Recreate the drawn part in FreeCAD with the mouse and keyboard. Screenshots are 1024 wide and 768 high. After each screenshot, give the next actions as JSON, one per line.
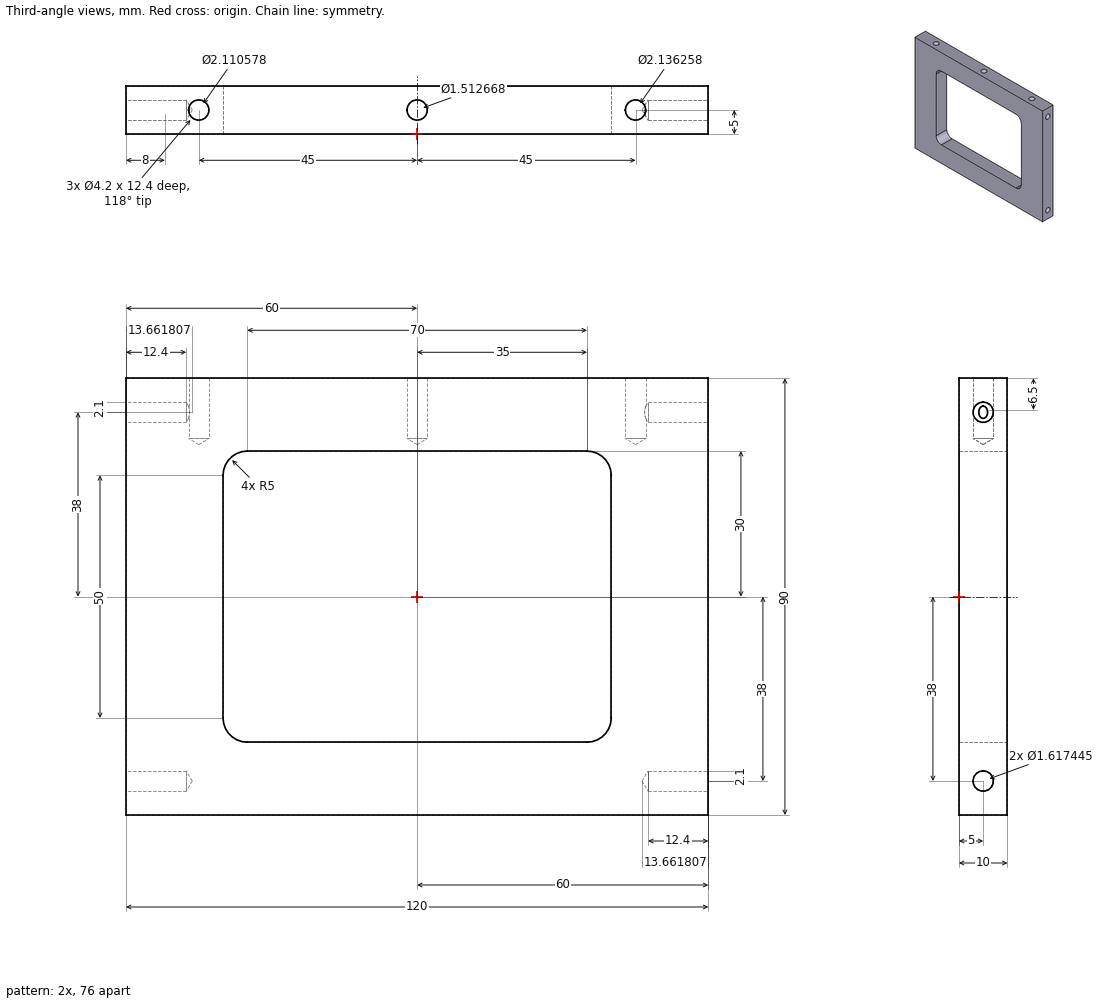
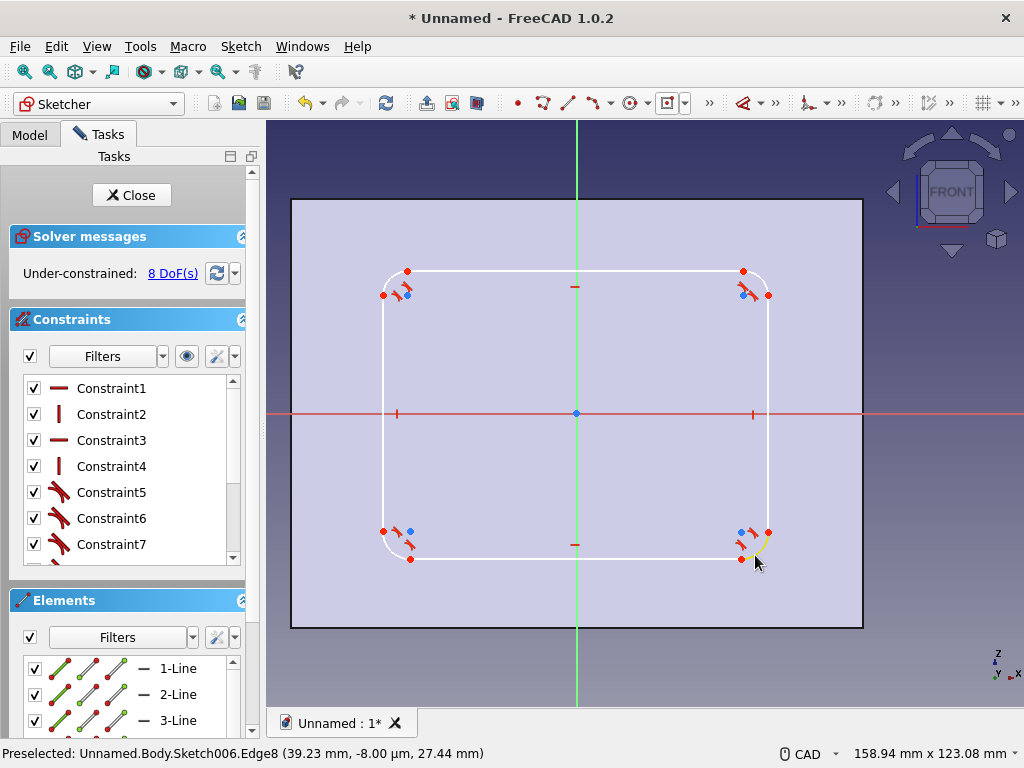
{"action": "left_click", "coordinate": [396, 274]}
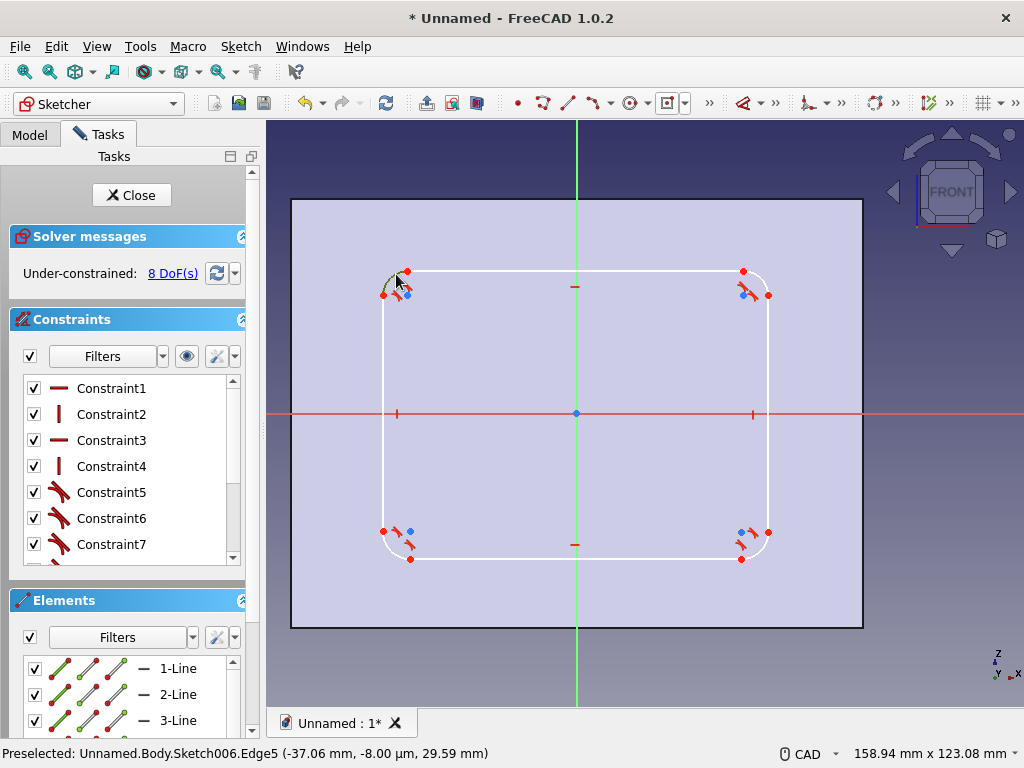
{"action": "left_click", "coordinate": [386, 544]}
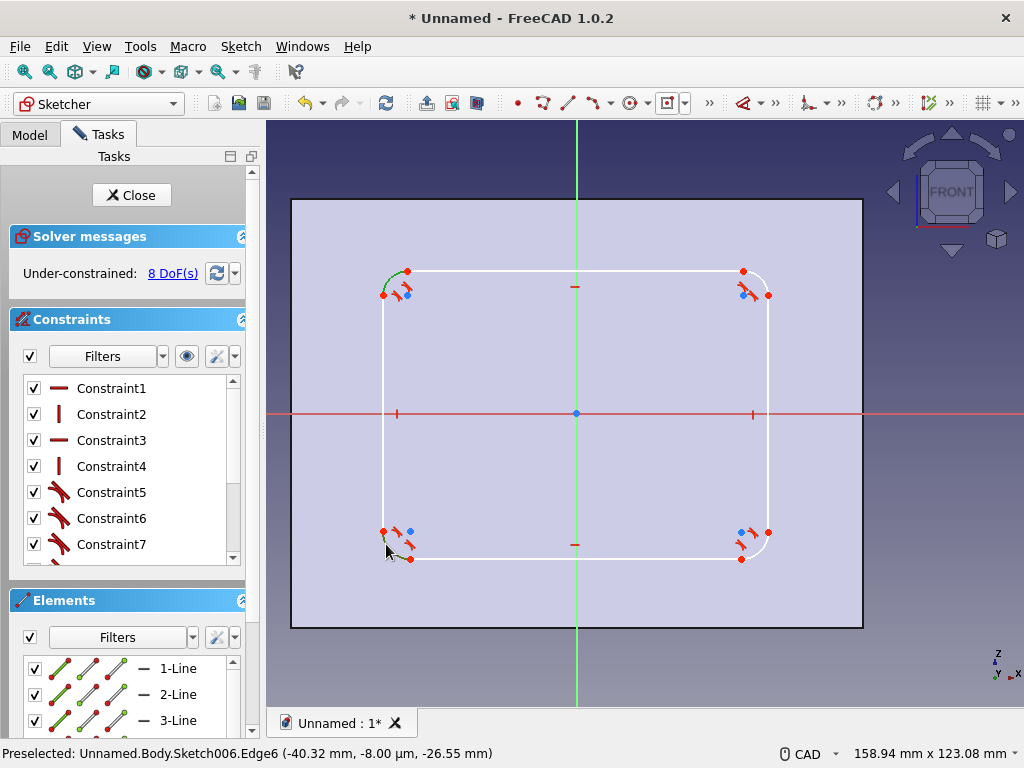
{"action": "left_click", "coordinate": [754, 556]}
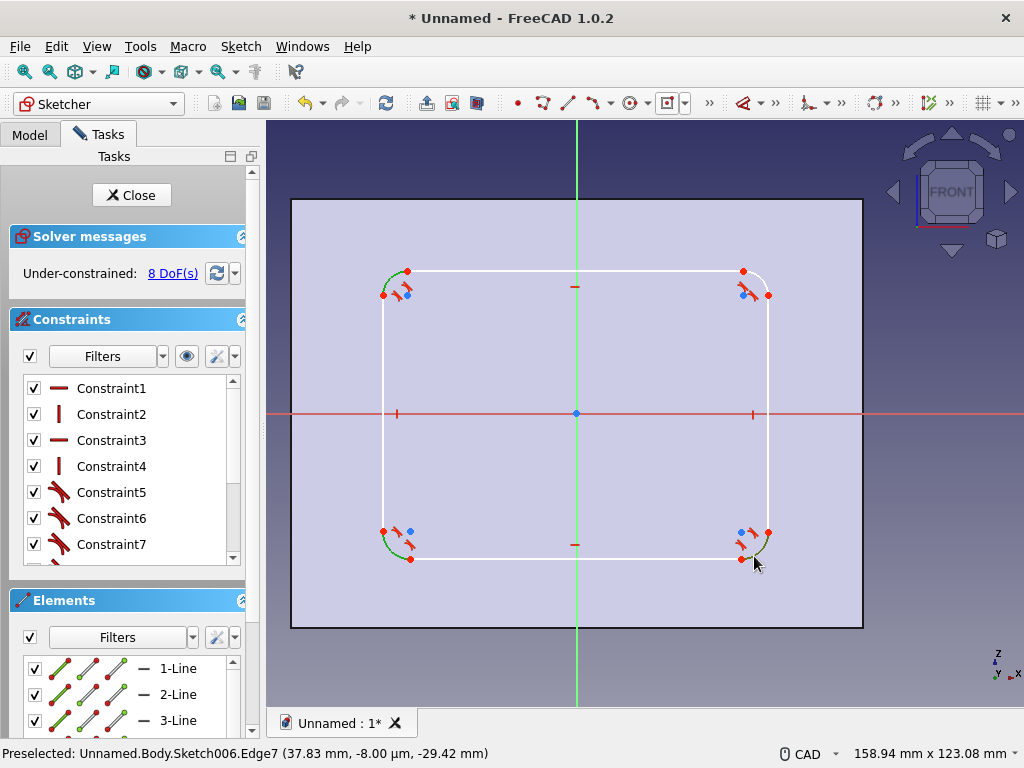
{"action": "left_click", "coordinate": [766, 285]}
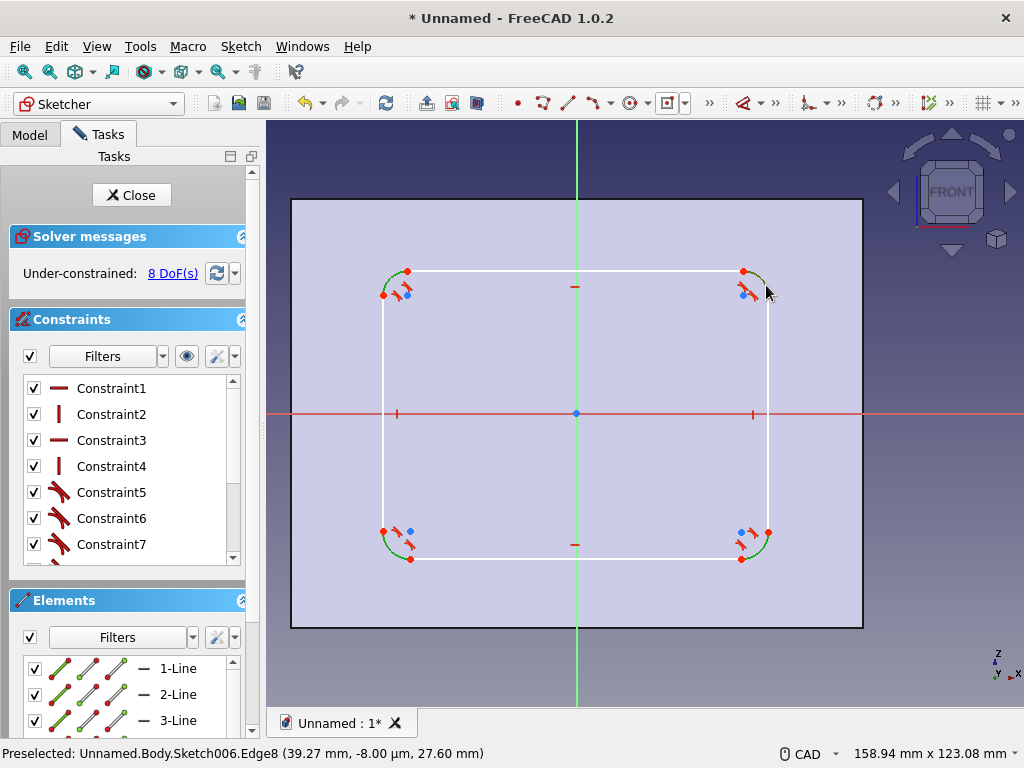
{"action": "key", "text": "e"}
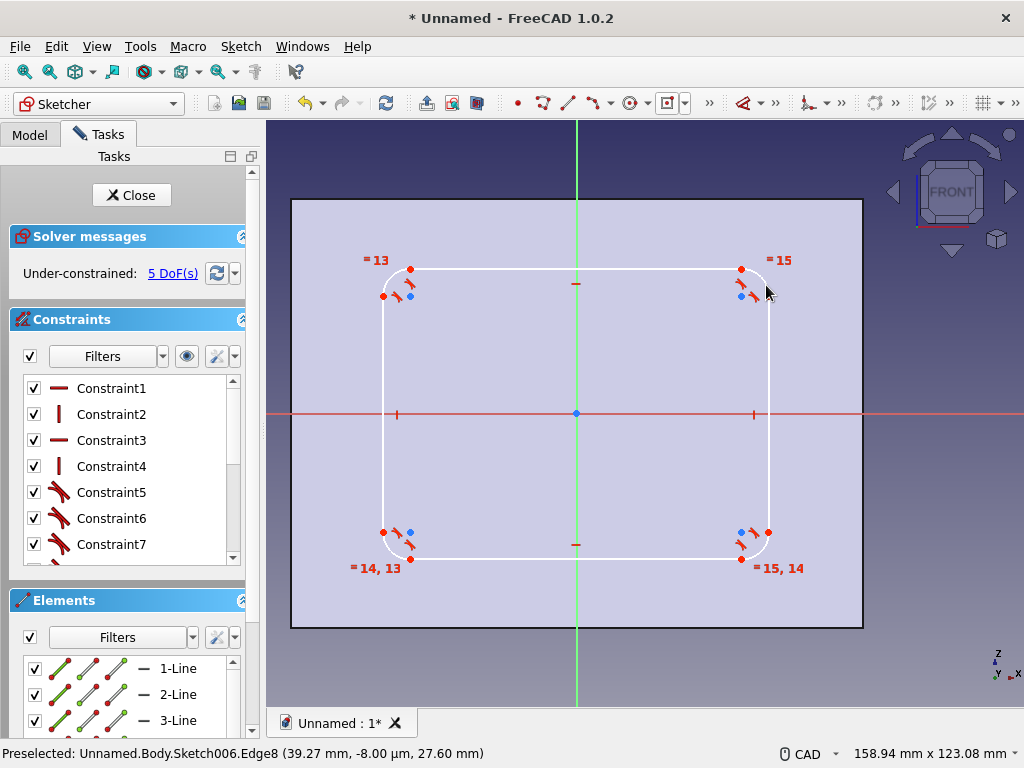
{"action": "left_click", "coordinate": [742, 104]}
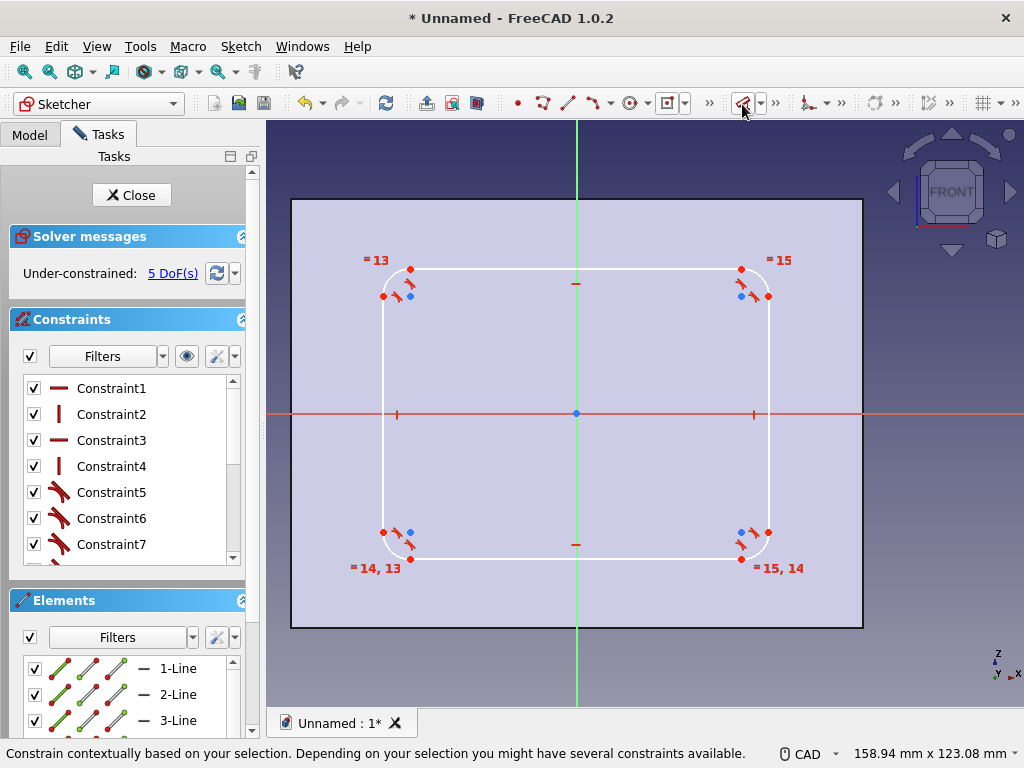
{"action": "scroll", "coordinate": [398, 272], "scroll_direction": "up", "scroll_amount": 3}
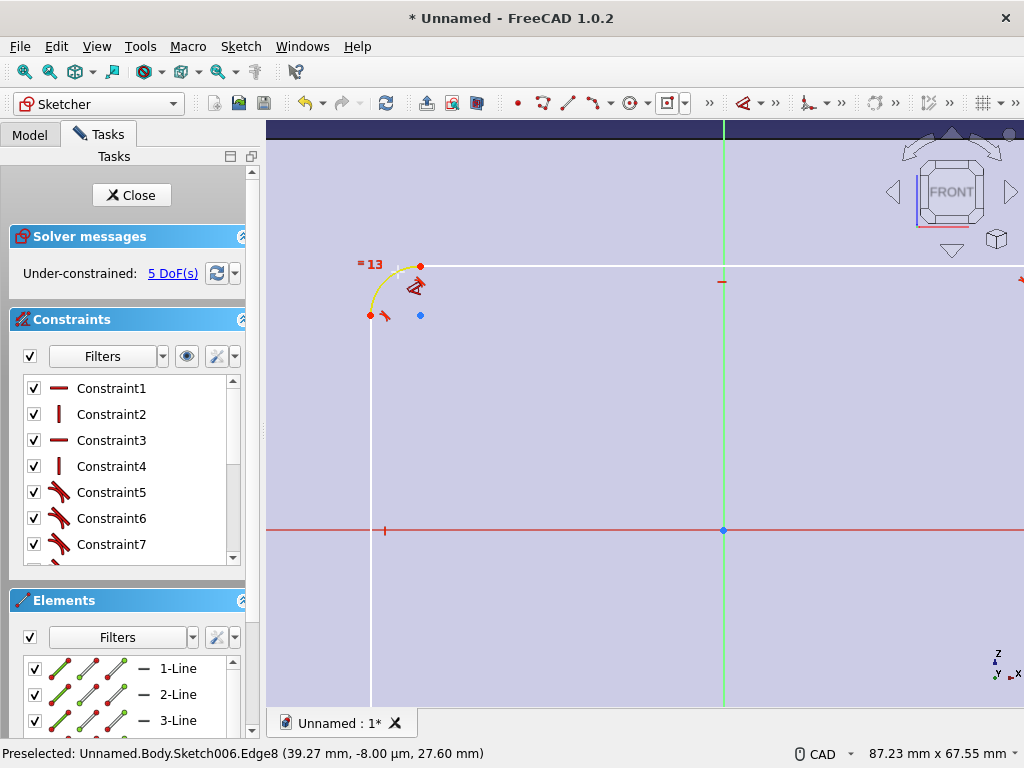
{"action": "left_click", "coordinate": [398, 272]}
{"action": "left_click", "coordinate": [383, 243]}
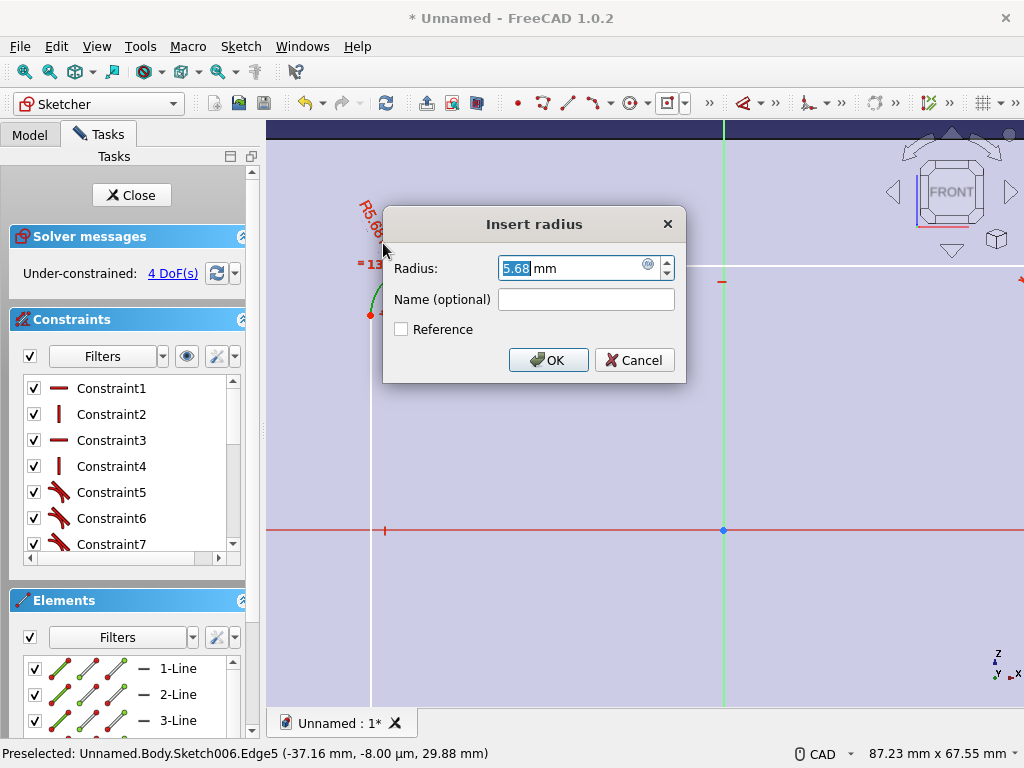
{"action": "type", "text": "5"}
{"action": "key", "text": "Return"}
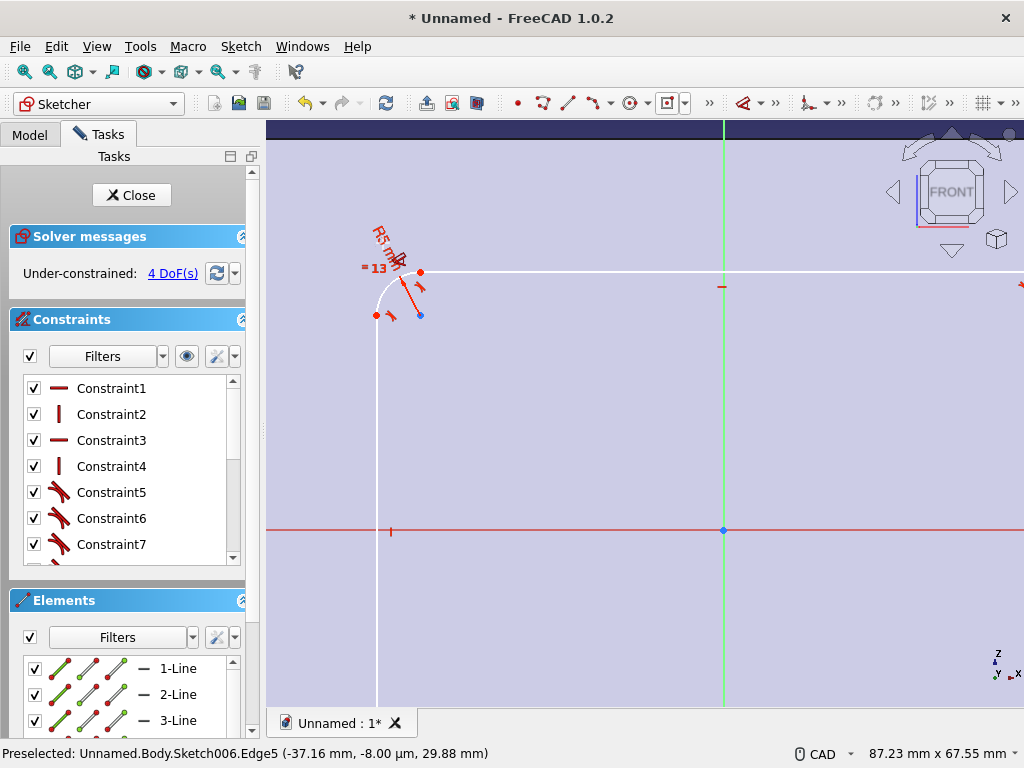
{"action": "left_click", "coordinate": [843, 272]}
{"action": "left_click", "coordinate": [640, 238]}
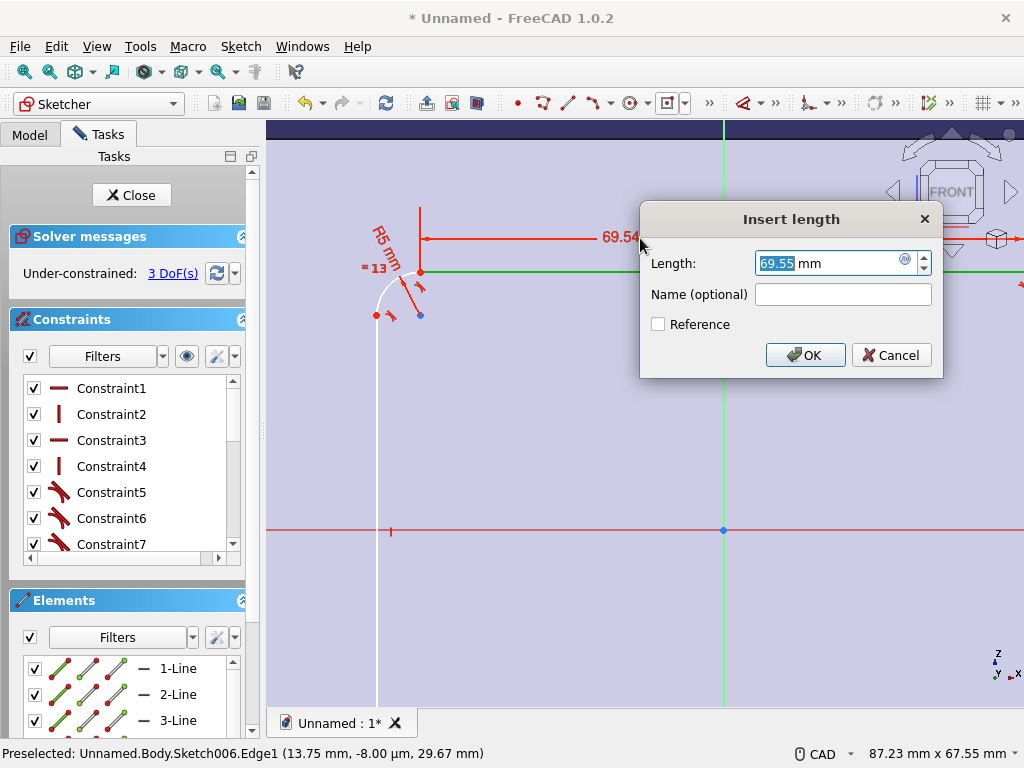
{"action": "type", "text": "70"}
{"action": "key", "text": "Return"}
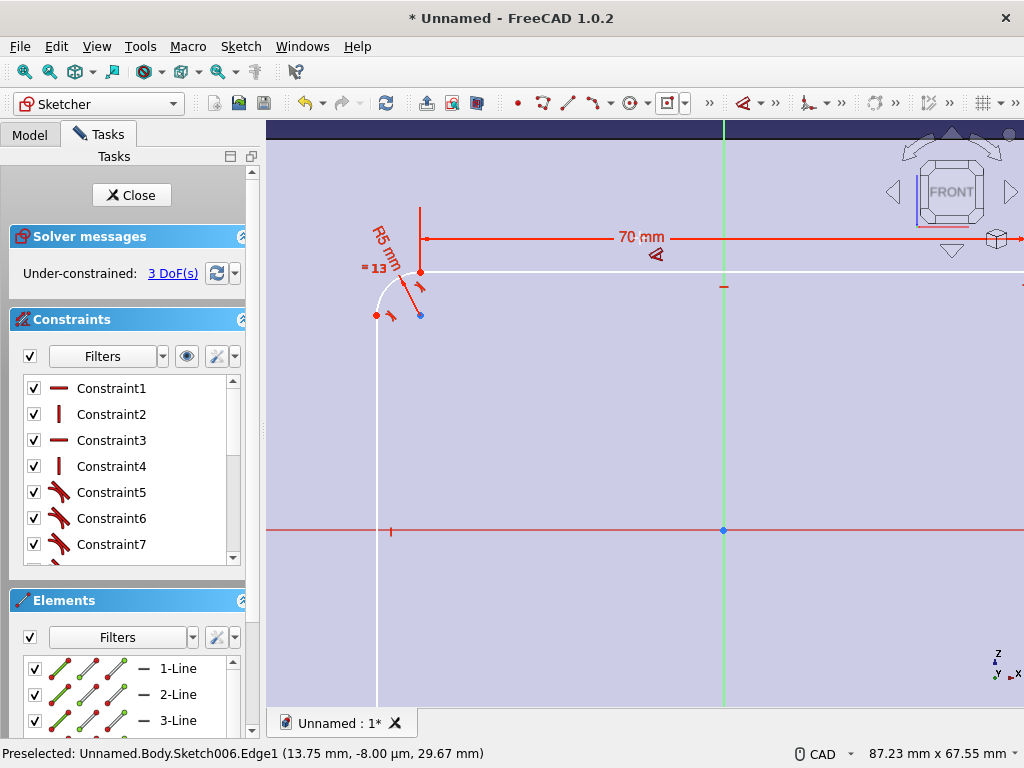
{"action": "left_click", "coordinate": [377, 445]}
{"action": "left_click", "coordinate": [343, 497]}